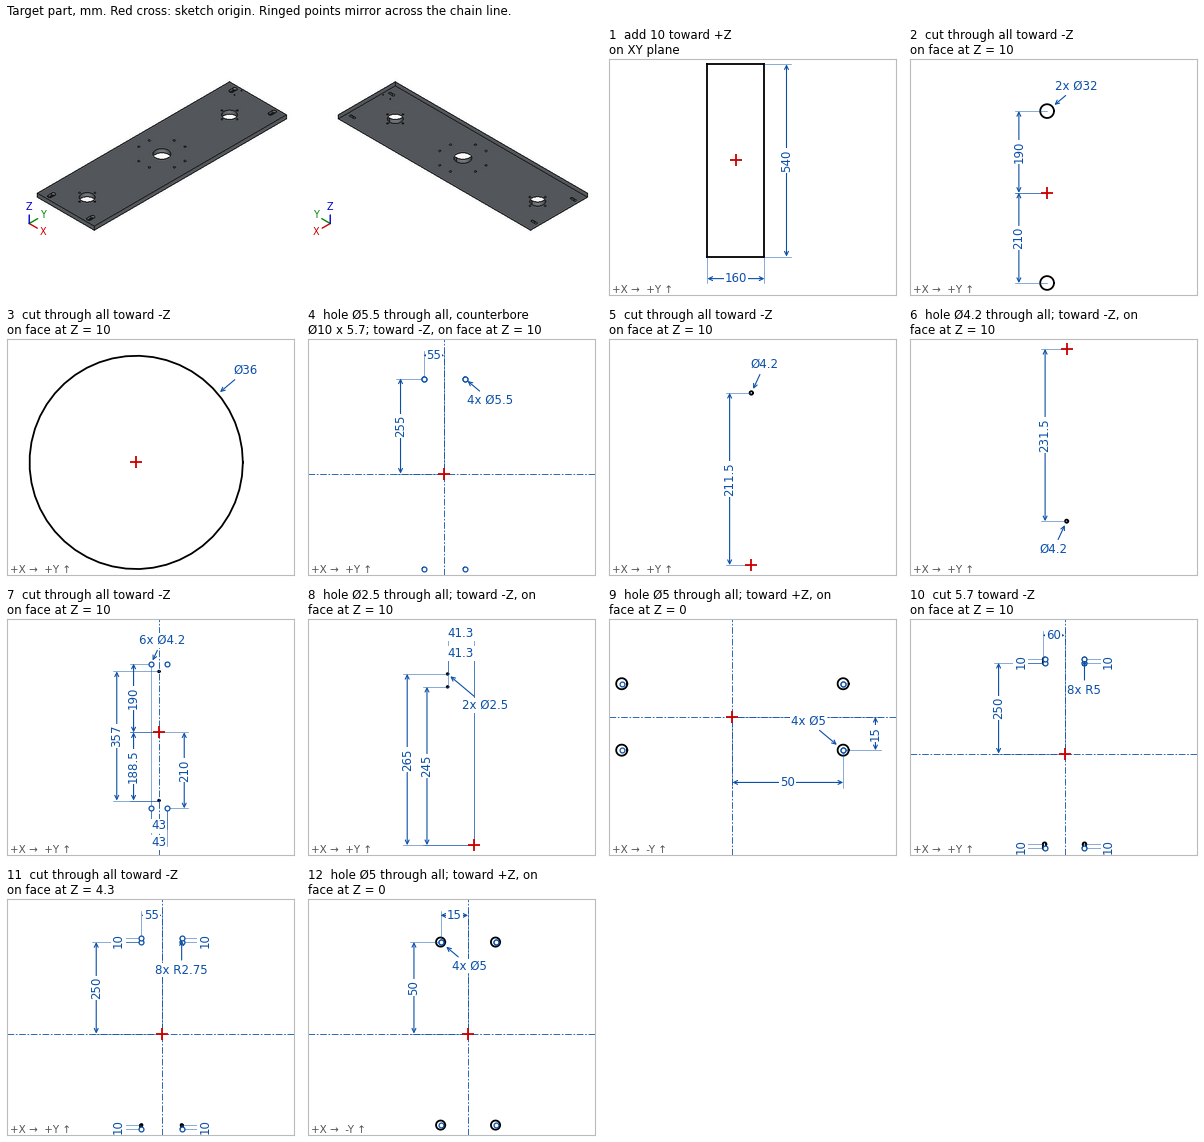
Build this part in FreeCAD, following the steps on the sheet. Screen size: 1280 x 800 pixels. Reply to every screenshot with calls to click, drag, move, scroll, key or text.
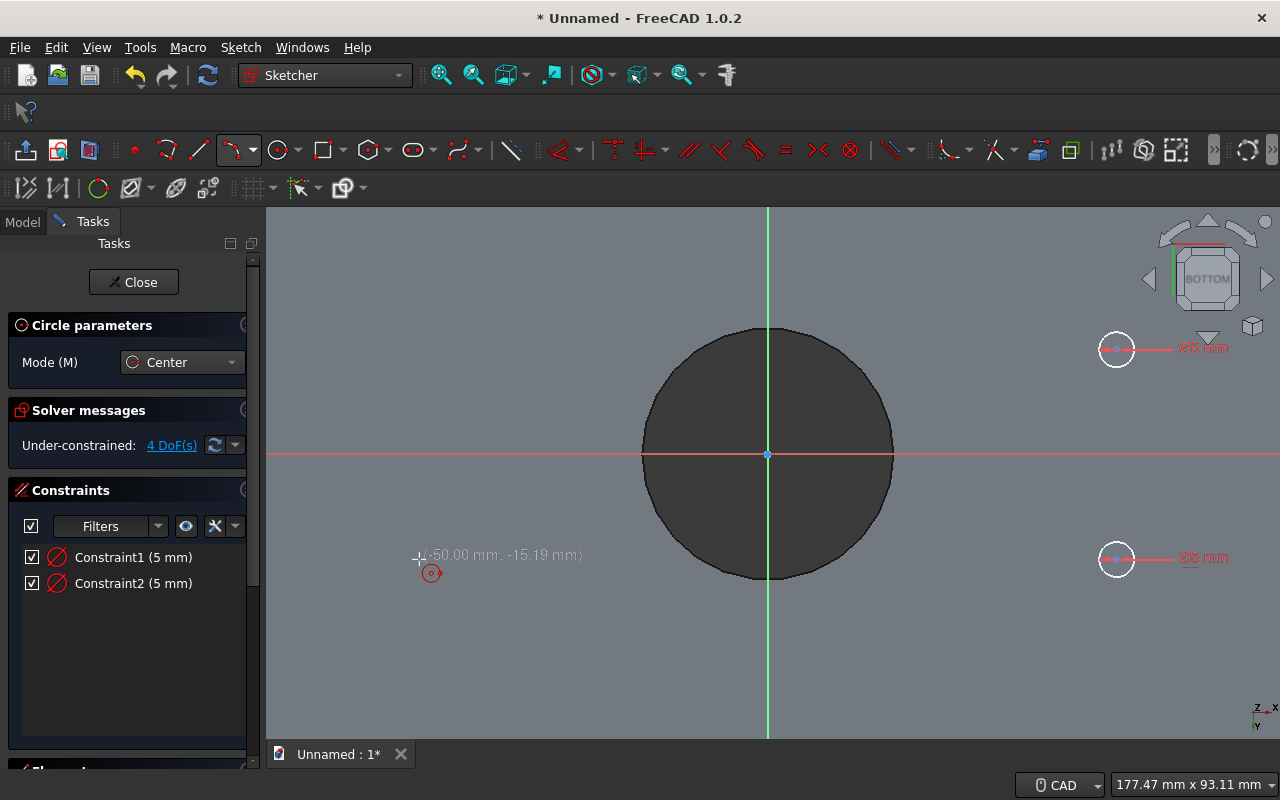
click(419, 558)
move(437, 540)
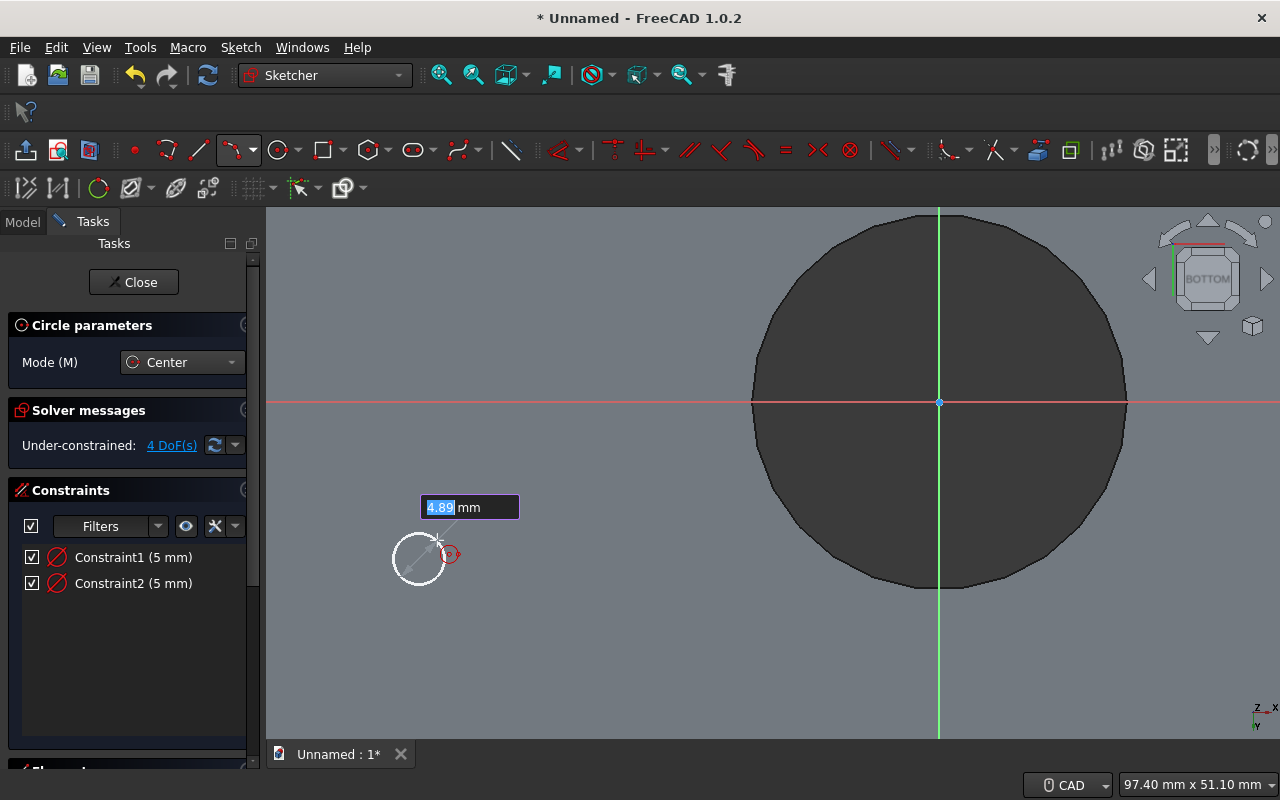
text(5)
key(Return)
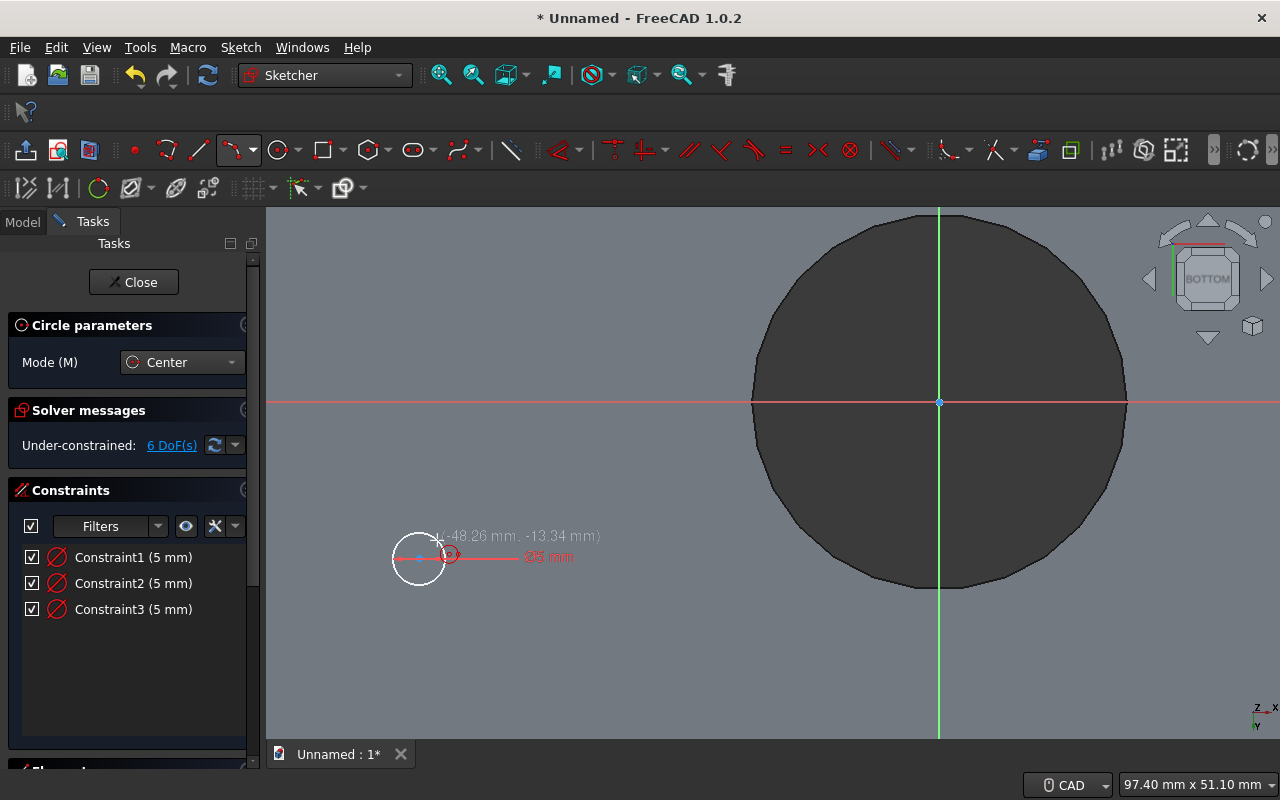
click(419, 246)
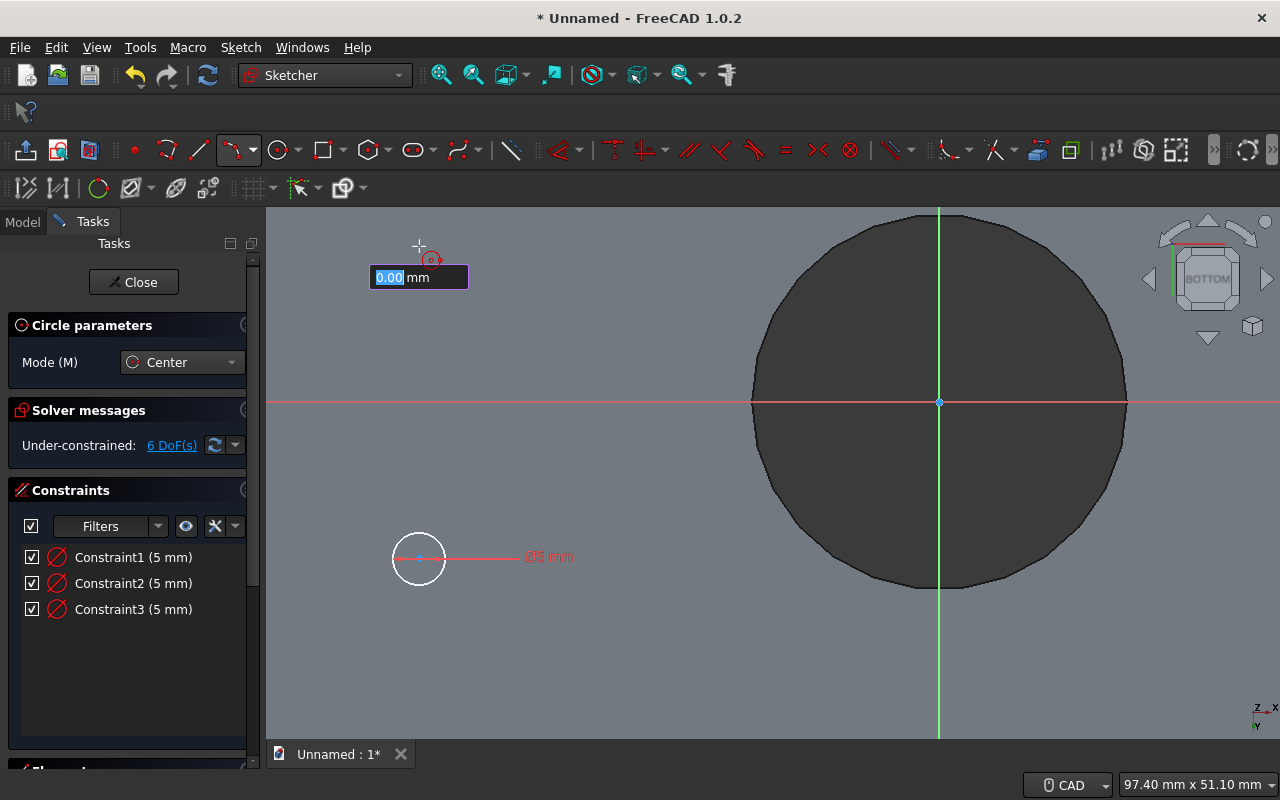
scroll(419, 559, down, 3)
move(429, 377)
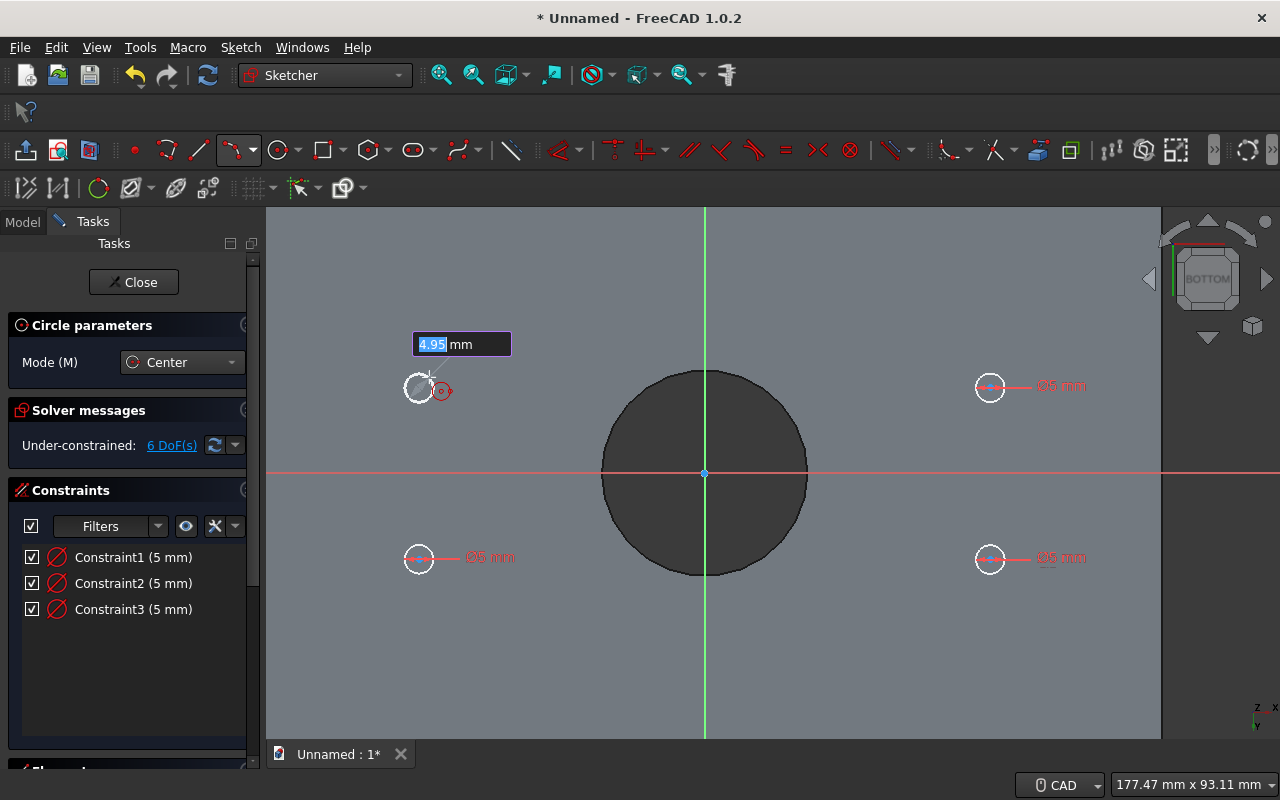
text(5)
key(Return)
key(Escape)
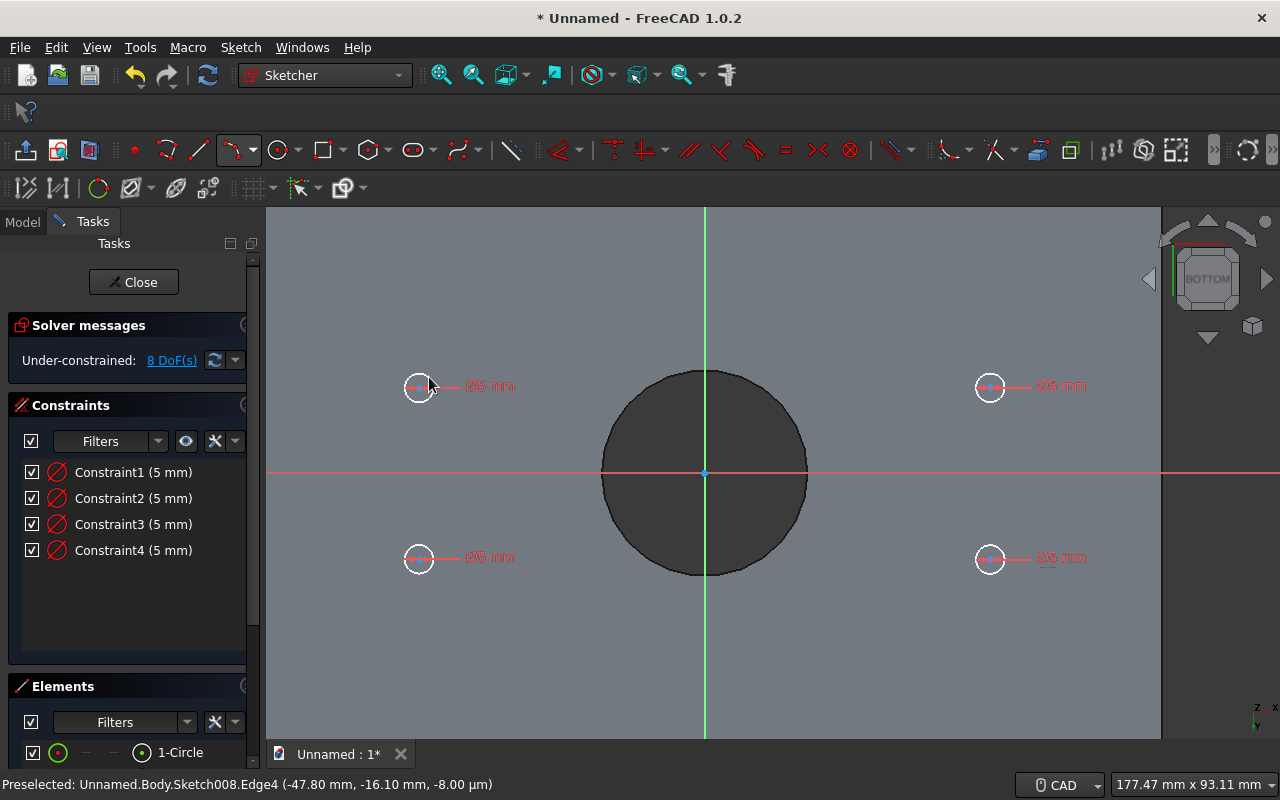
click(990, 560)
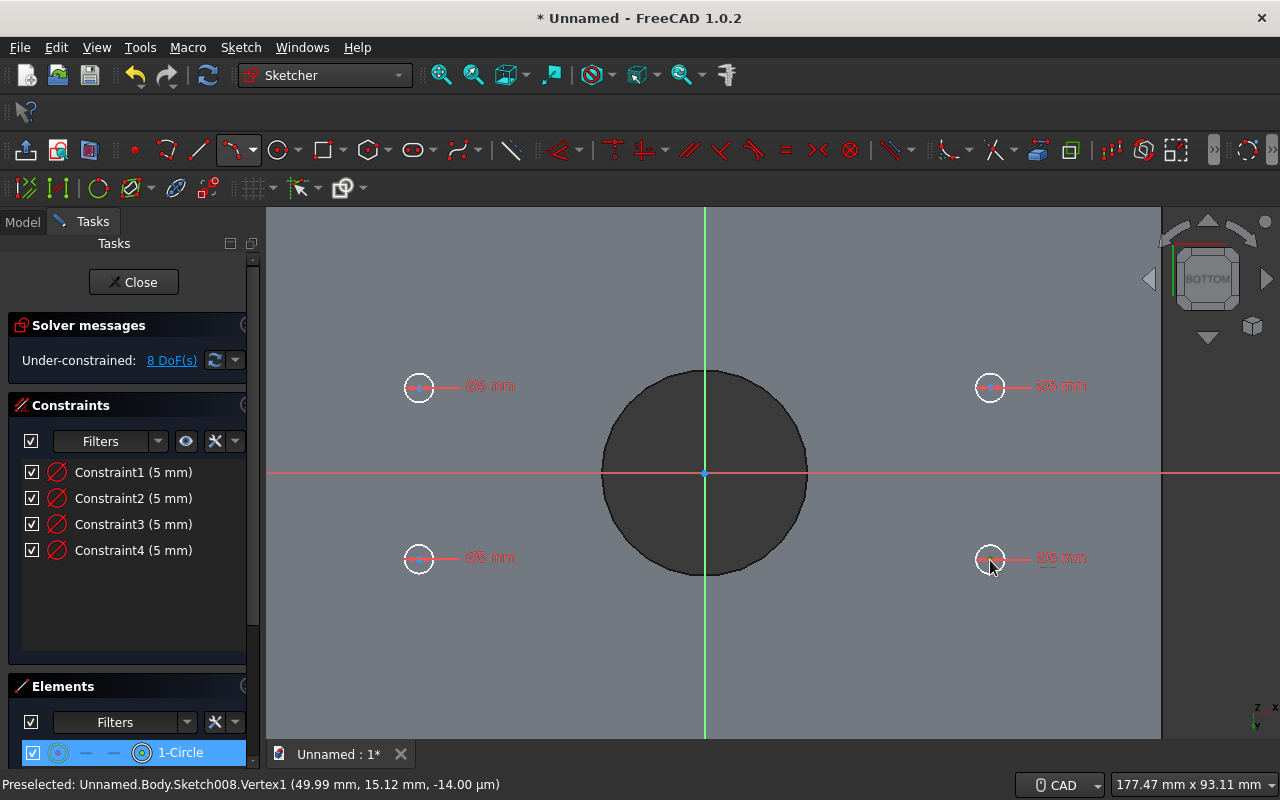
click(990, 388)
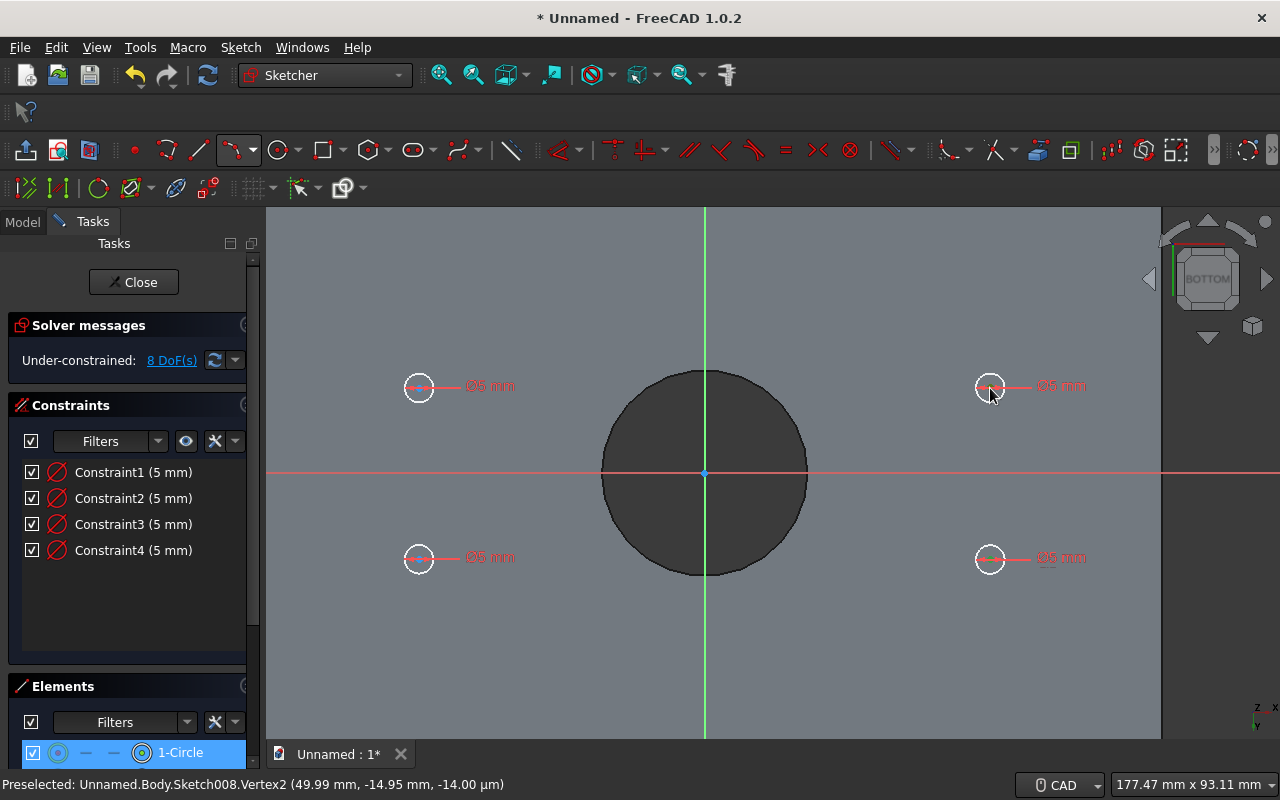
click(353, 473)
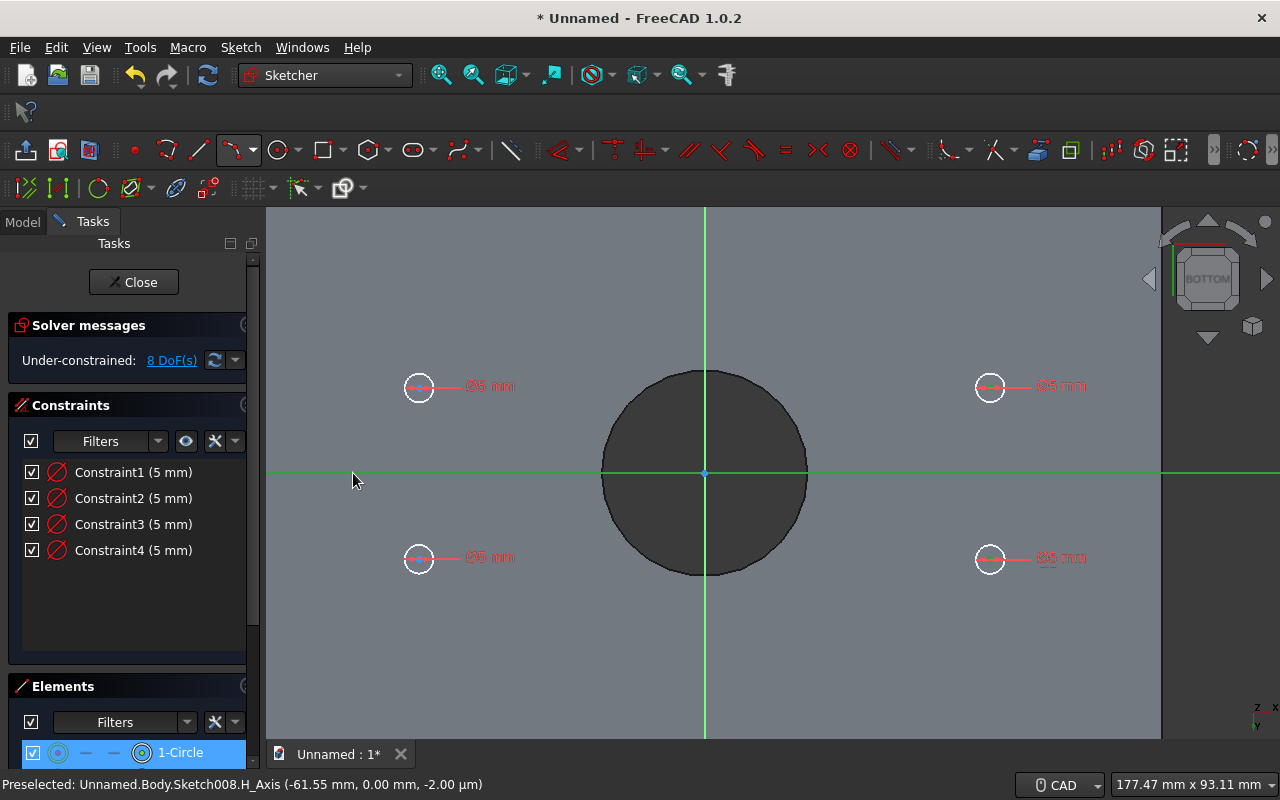
click(818, 150)